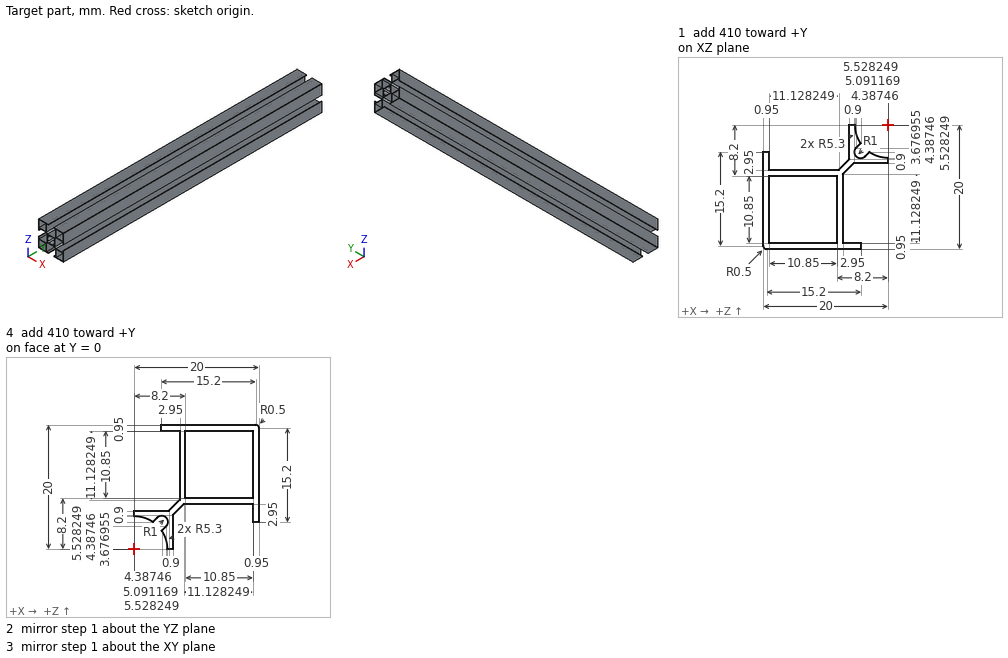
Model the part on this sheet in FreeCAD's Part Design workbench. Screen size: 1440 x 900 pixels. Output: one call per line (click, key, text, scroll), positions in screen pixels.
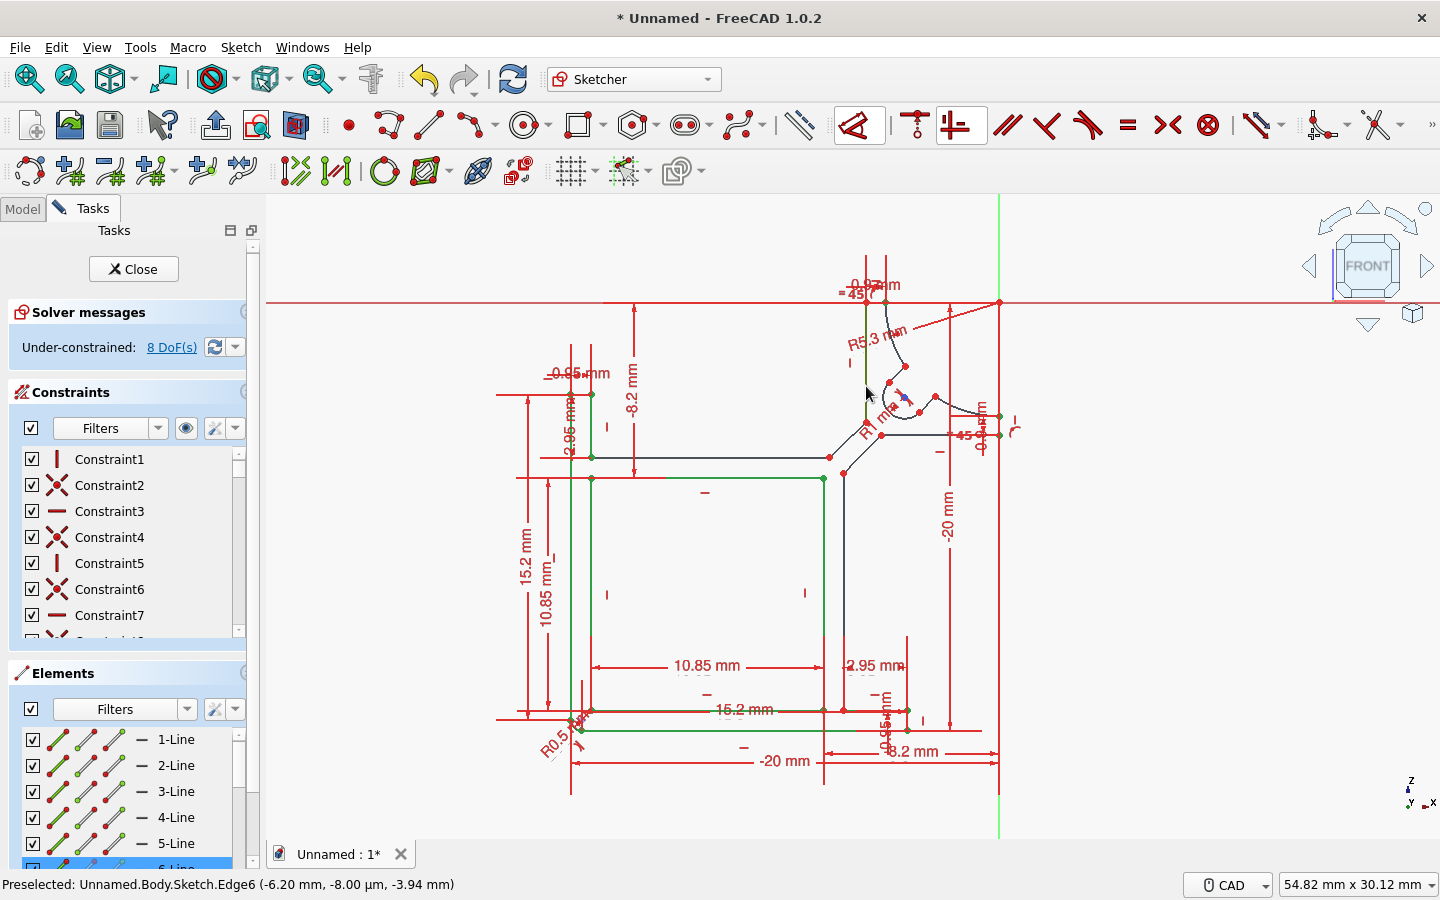
click(880, 126)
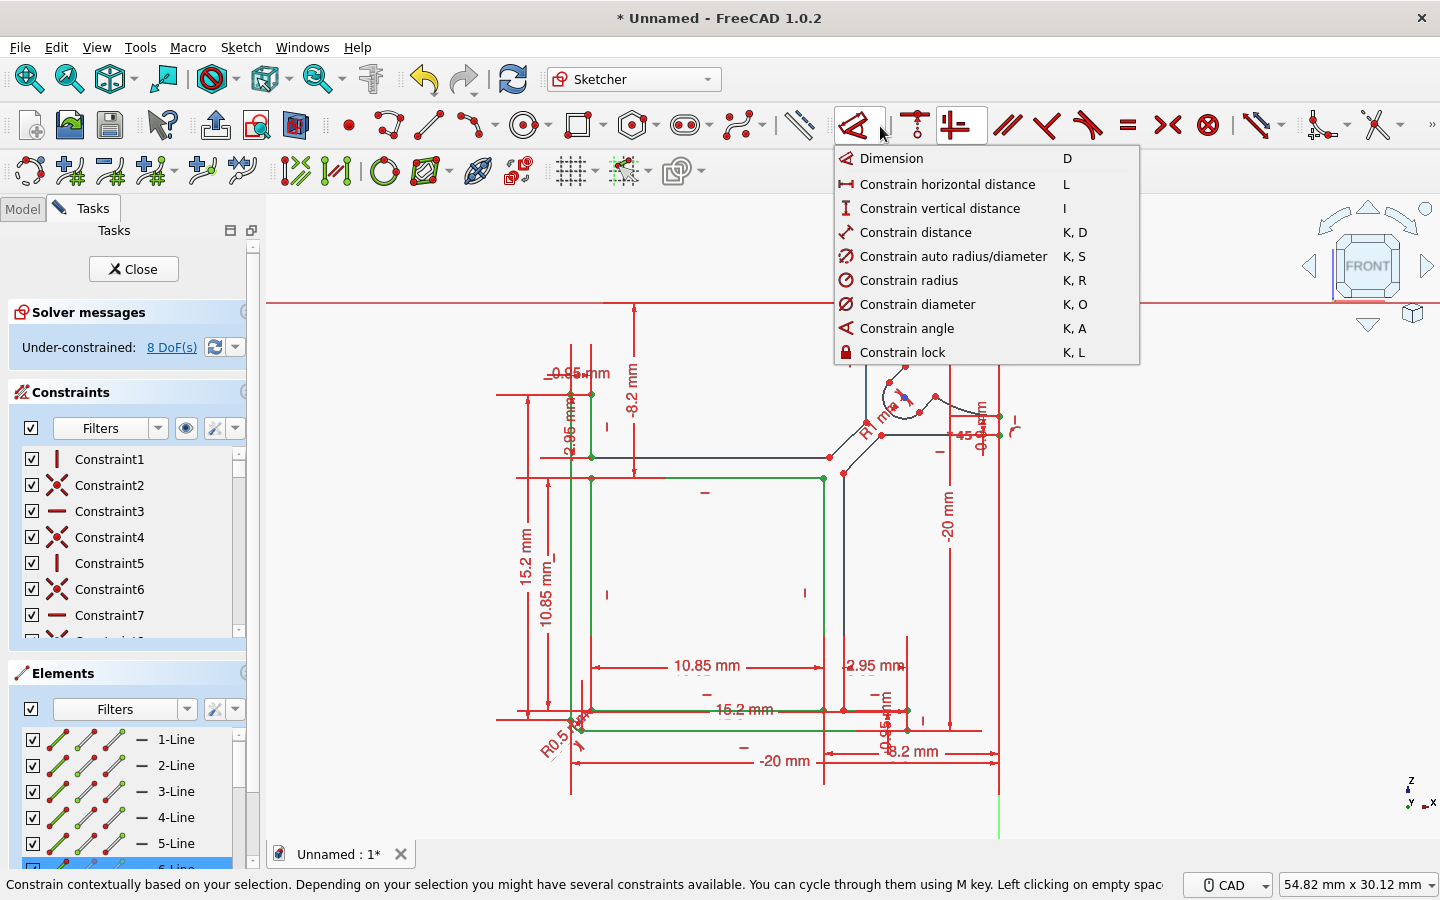
click(987, 208)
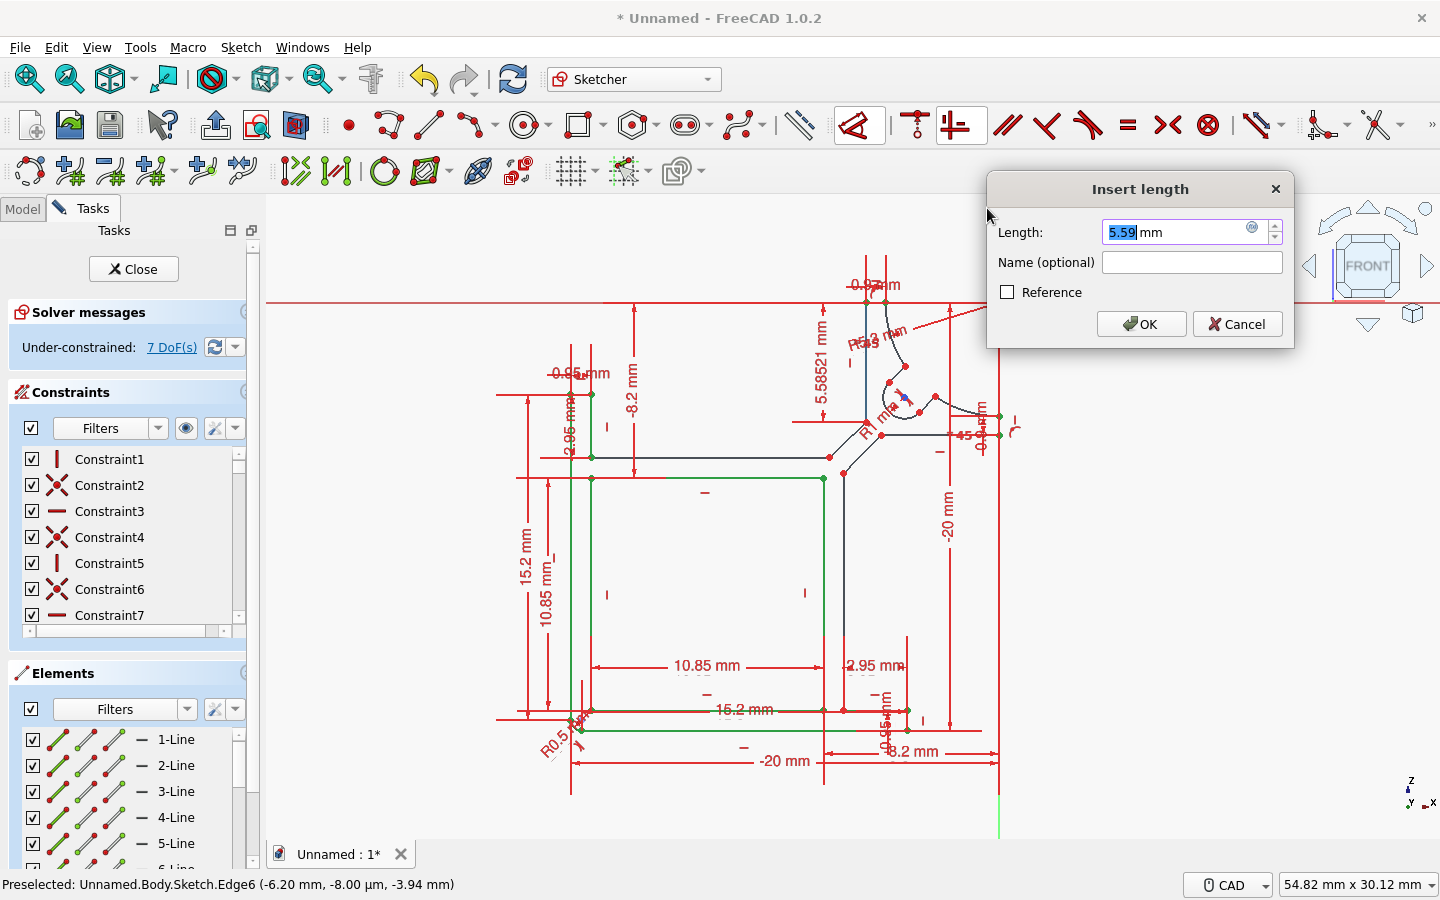
text(5.528249)
key(Return)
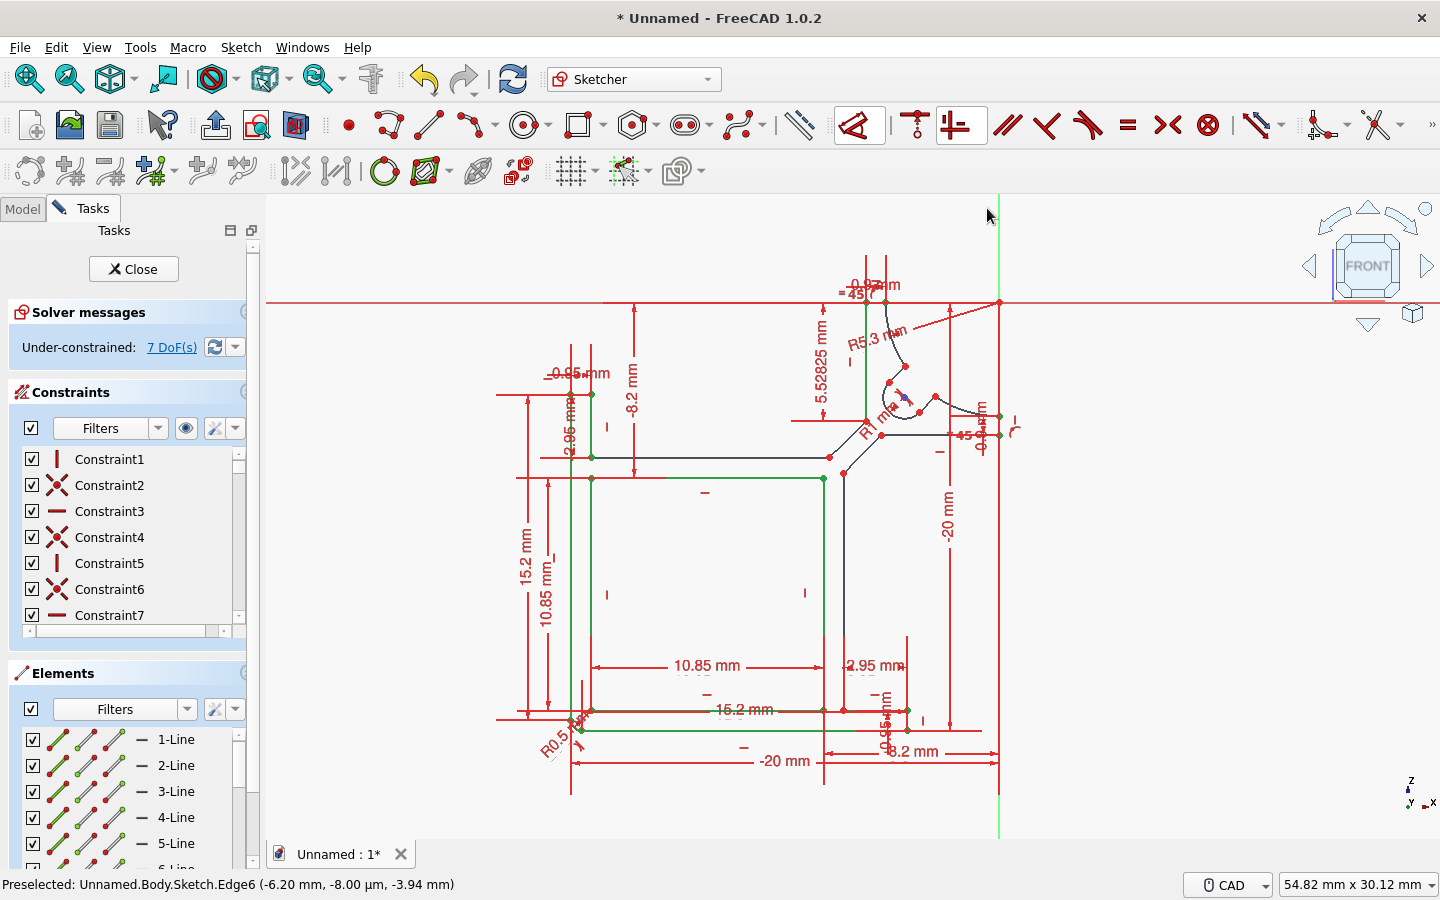
click(916, 435)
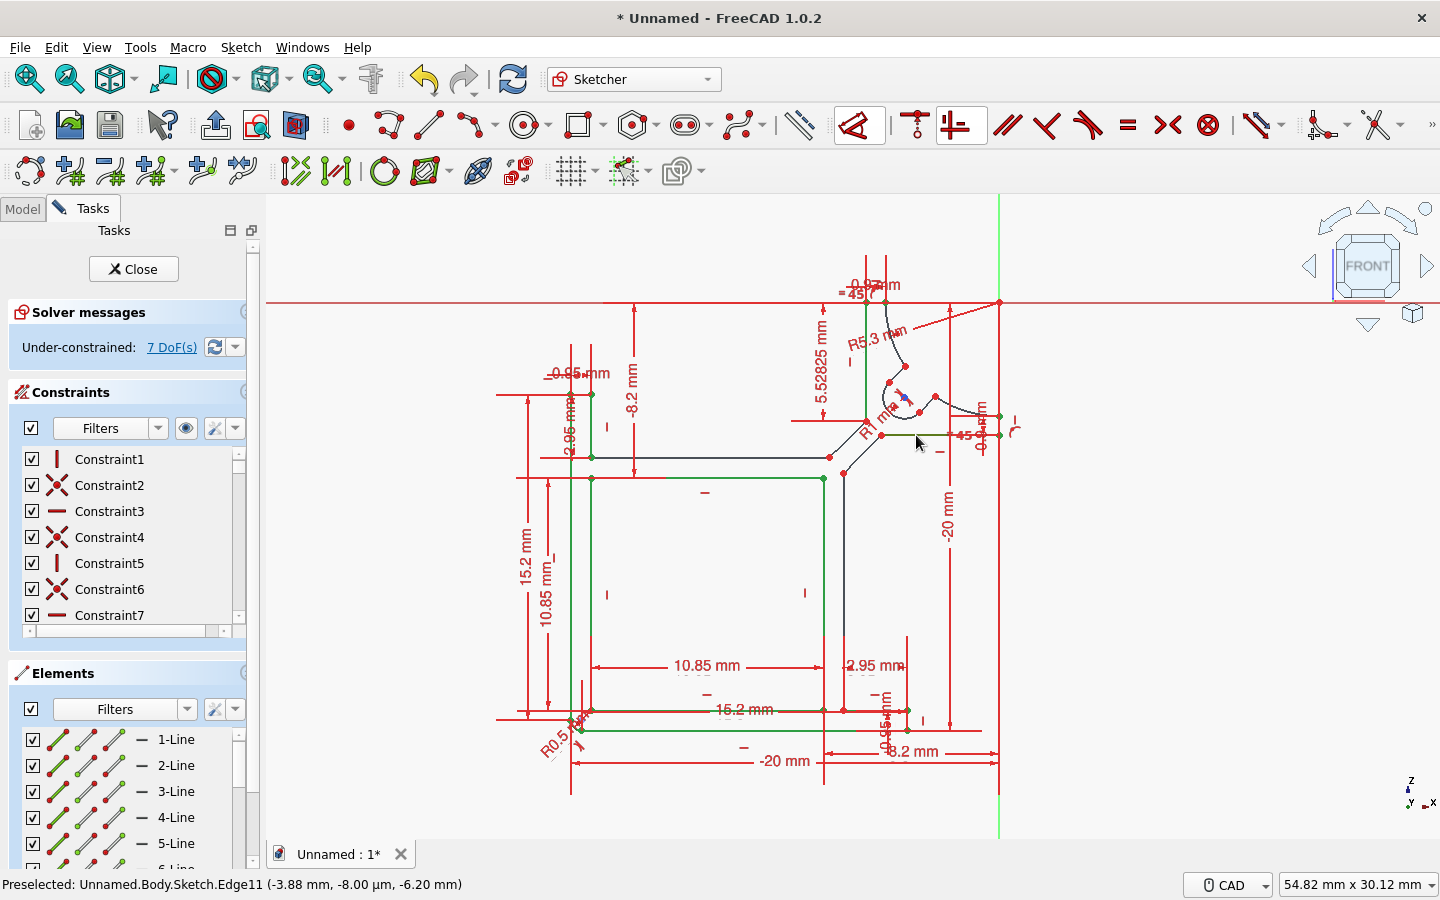
key(l)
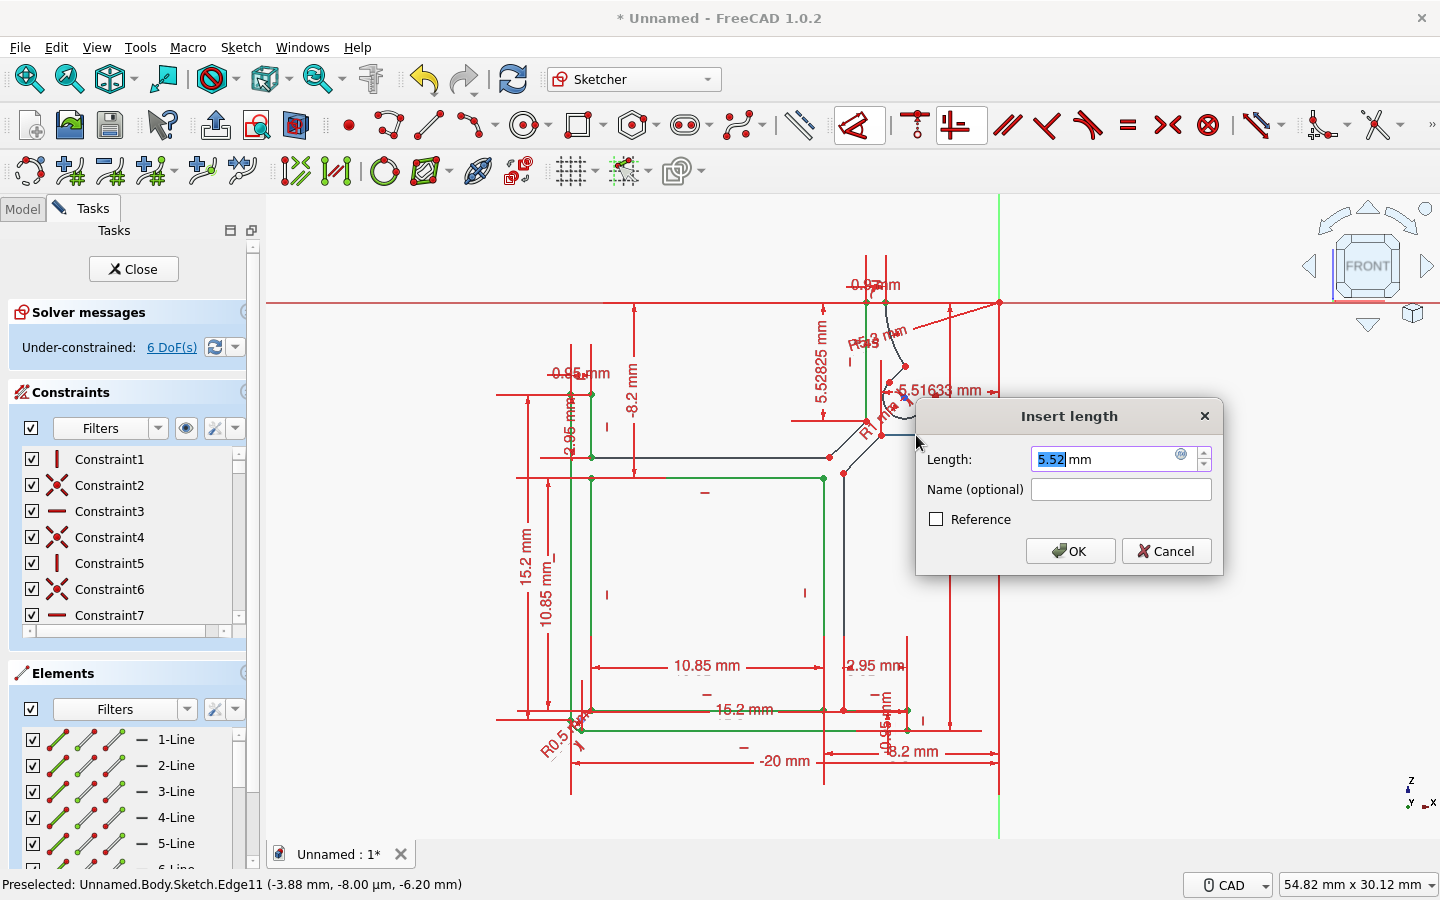
text(5.528249)
key(Return)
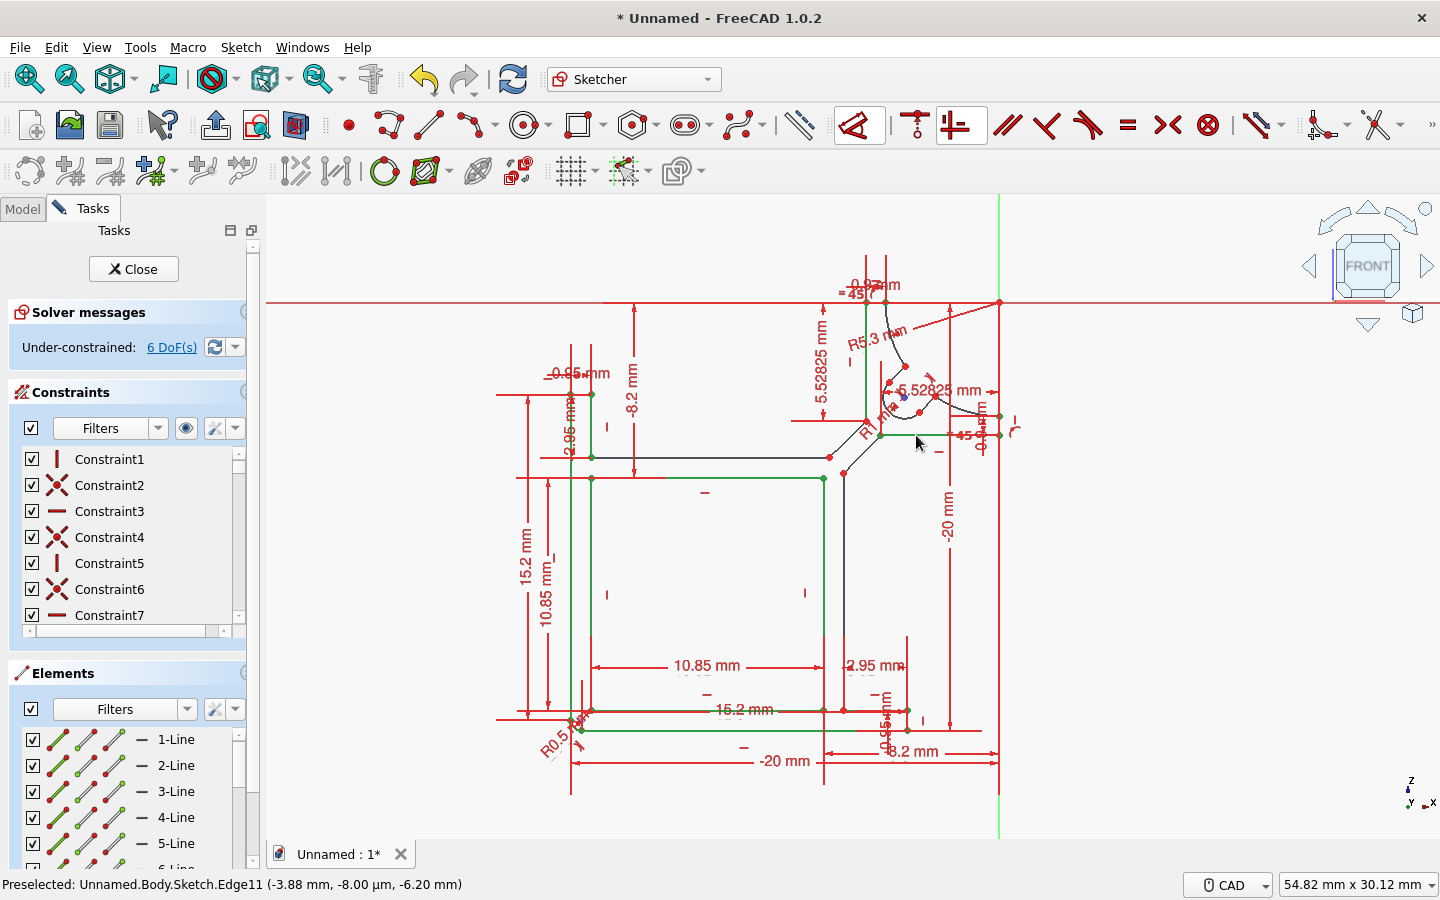
click(905, 366)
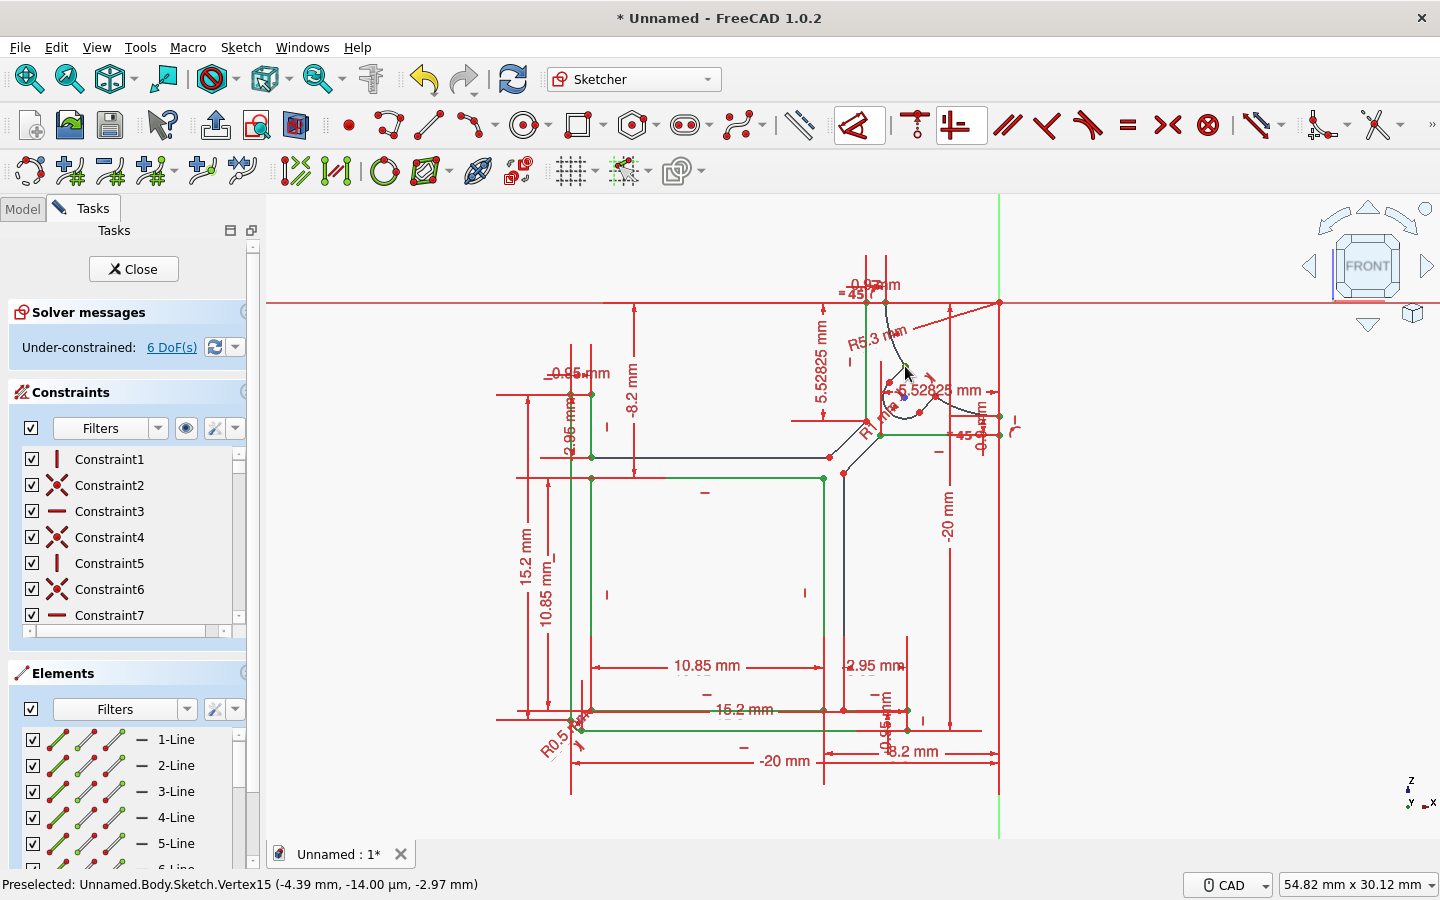
key(l)